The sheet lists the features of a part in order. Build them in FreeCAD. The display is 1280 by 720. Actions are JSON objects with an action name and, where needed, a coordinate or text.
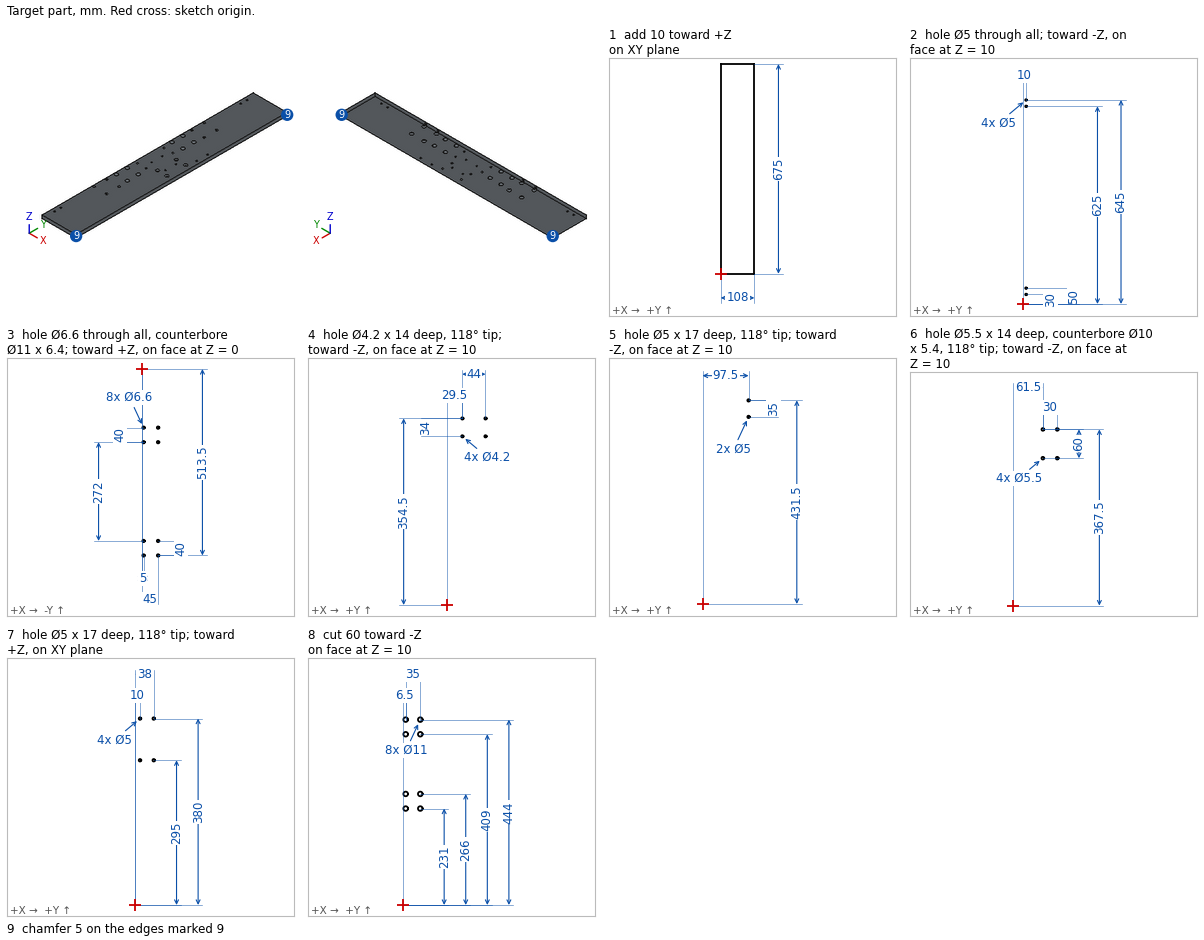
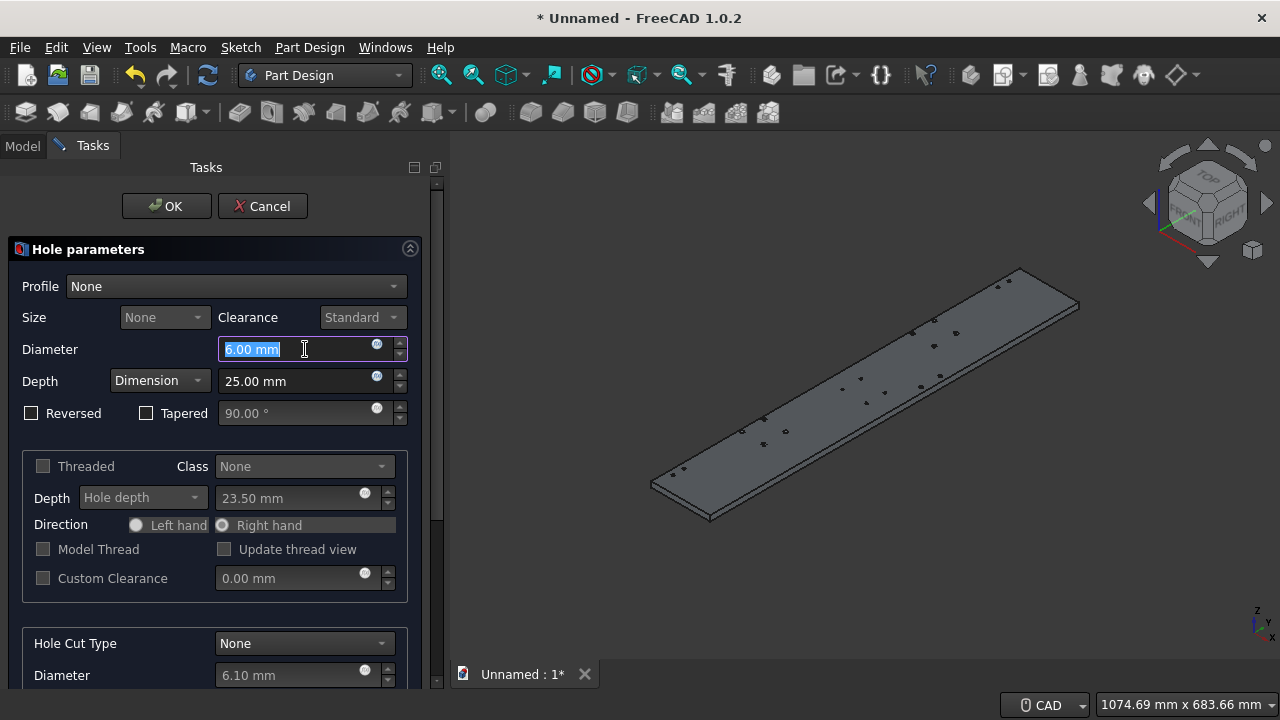
{"action": "type", "text": "5"}
{"action": "key", "text": "Tab"}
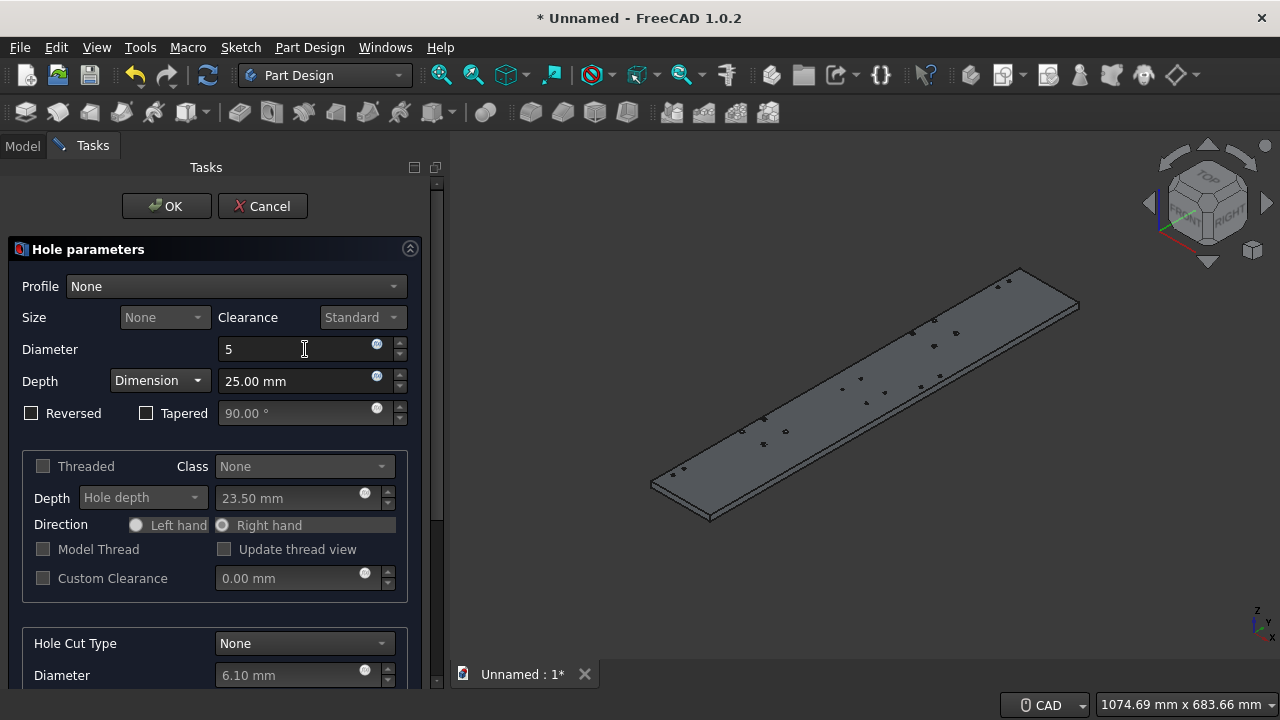
{"action": "triple_click", "coordinate": [305, 381]}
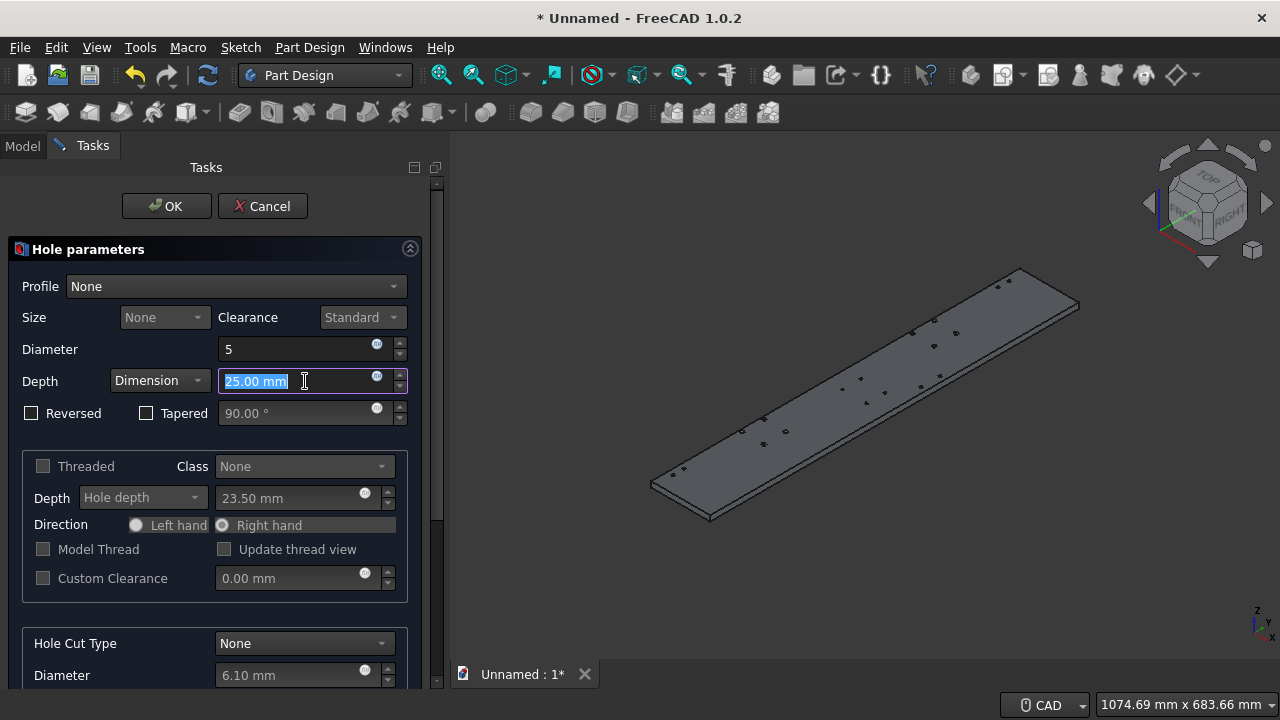
{"action": "type", "text": "17"}
{"action": "key", "text": "Tab"}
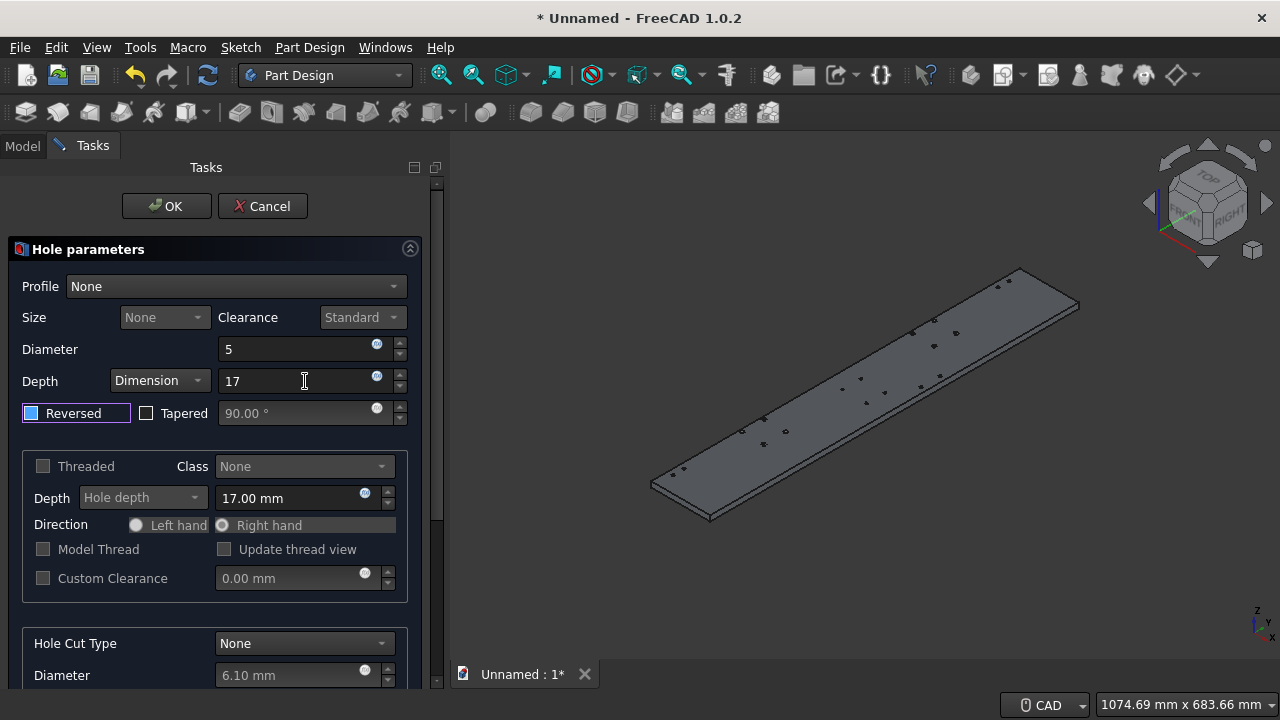
{"action": "left_click", "coordinate": [167, 206]}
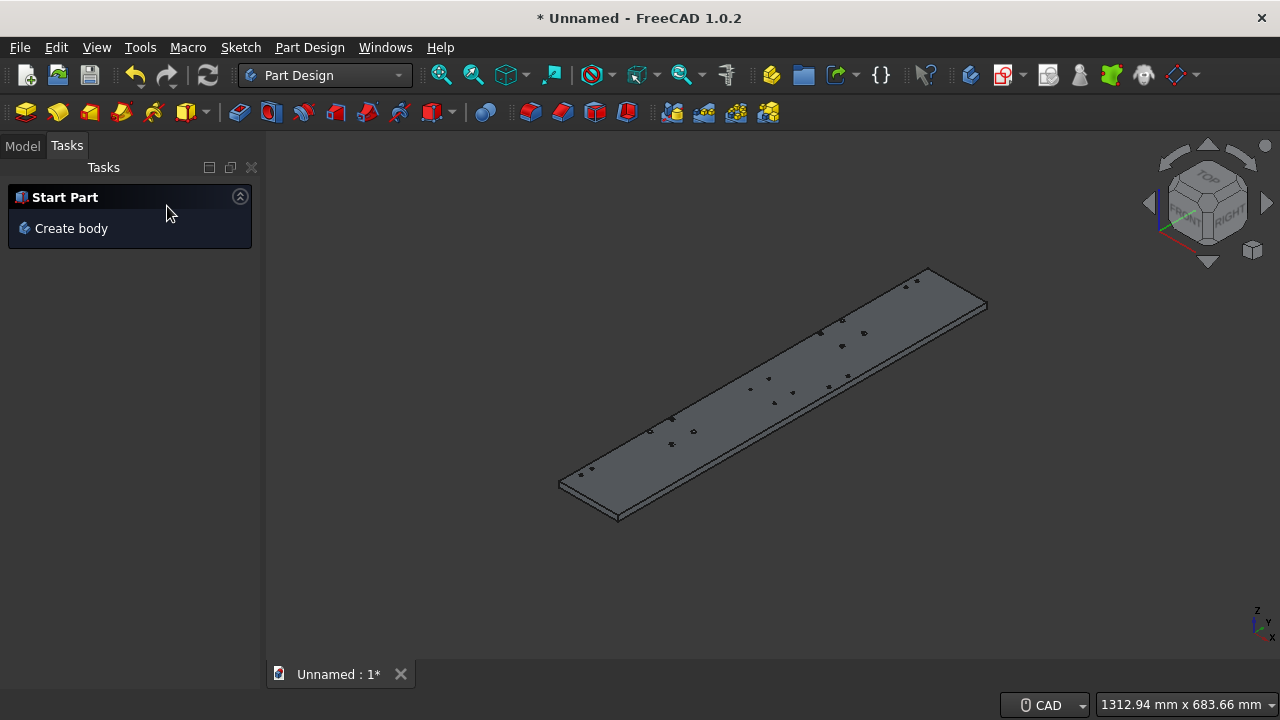
{"action": "left_click", "coordinate": [931, 300]}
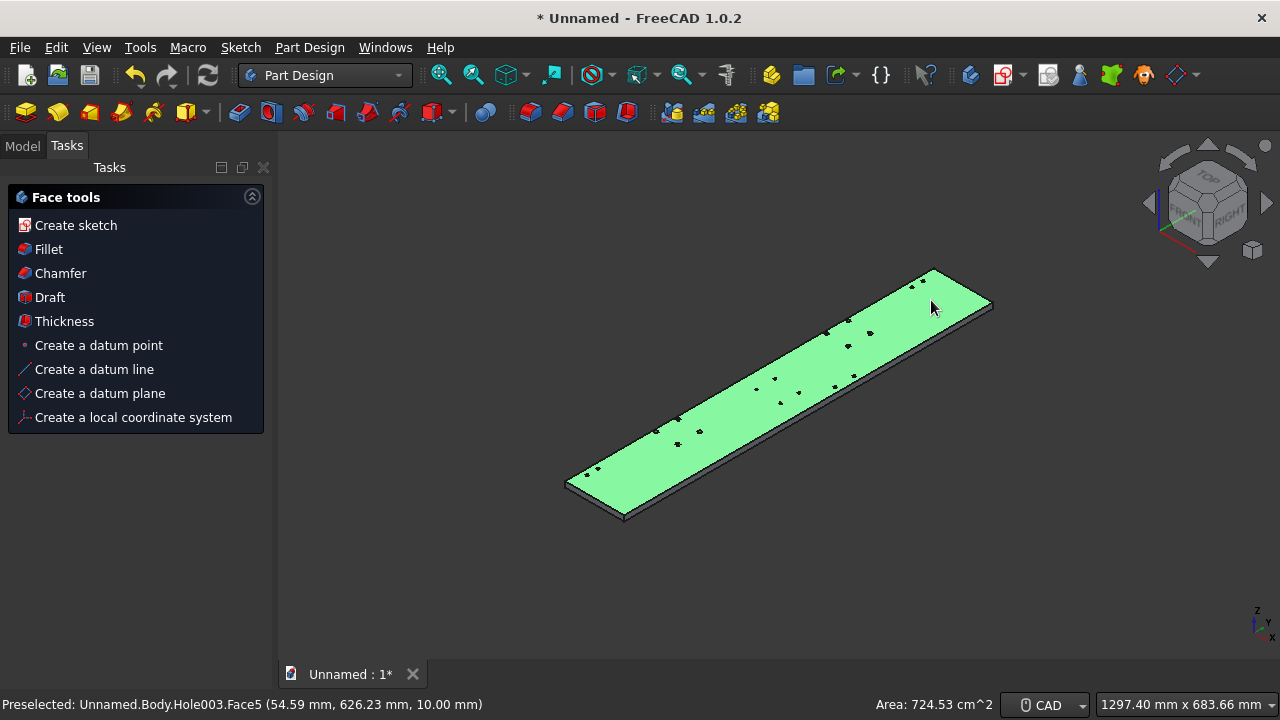
{"action": "left_click", "coordinate": [1004, 76]}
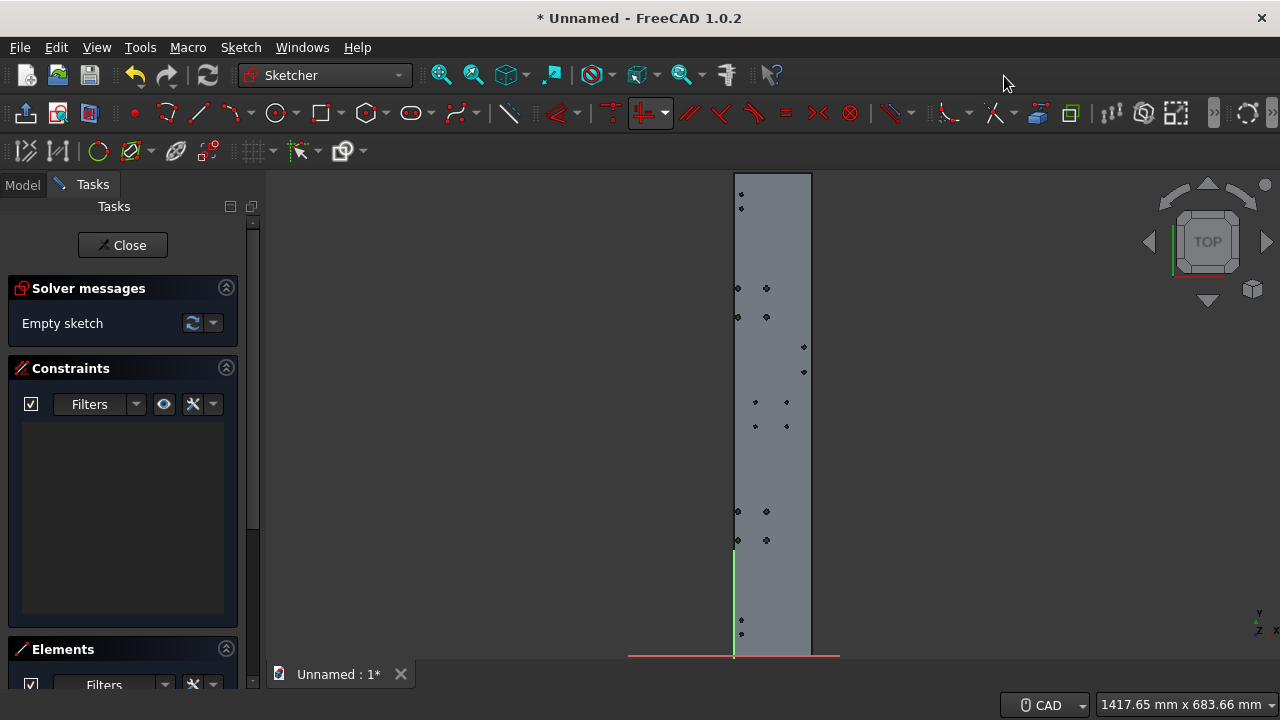
{"action": "scroll", "coordinate": [806, 414], "scroll_direction": "up", "scroll_amount": 9}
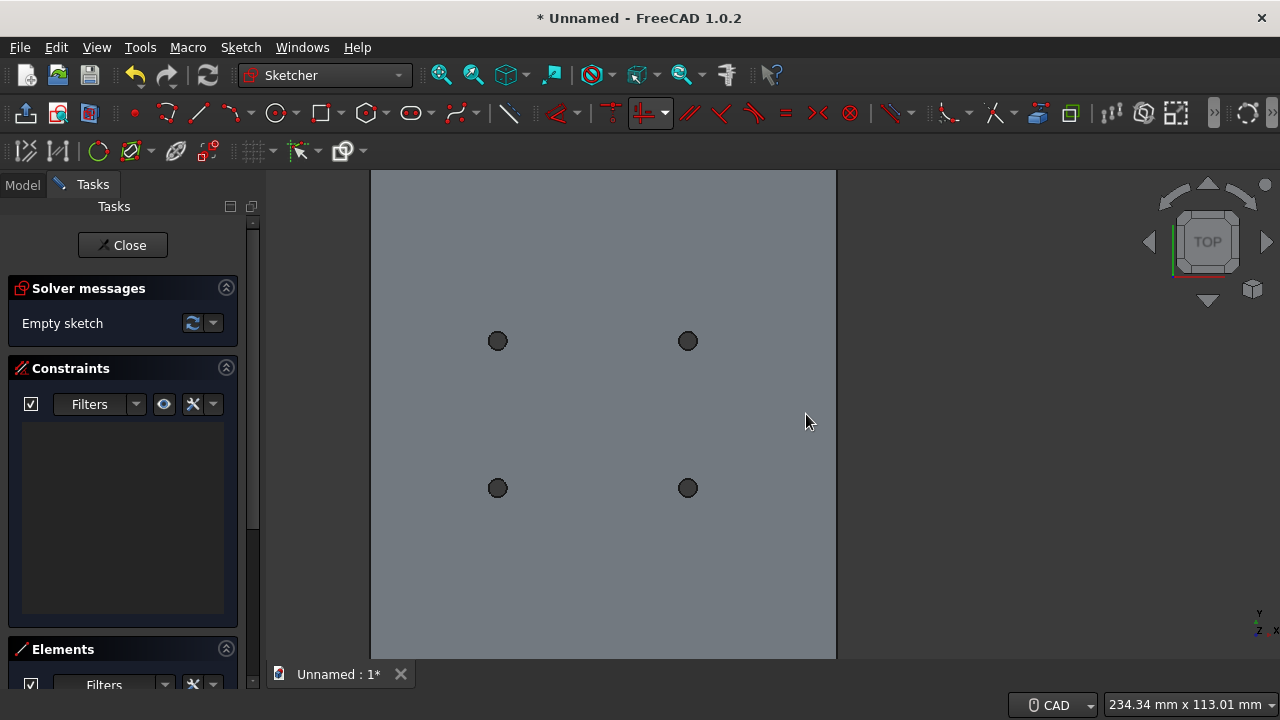
{"action": "left_click", "coordinate": [276, 114]}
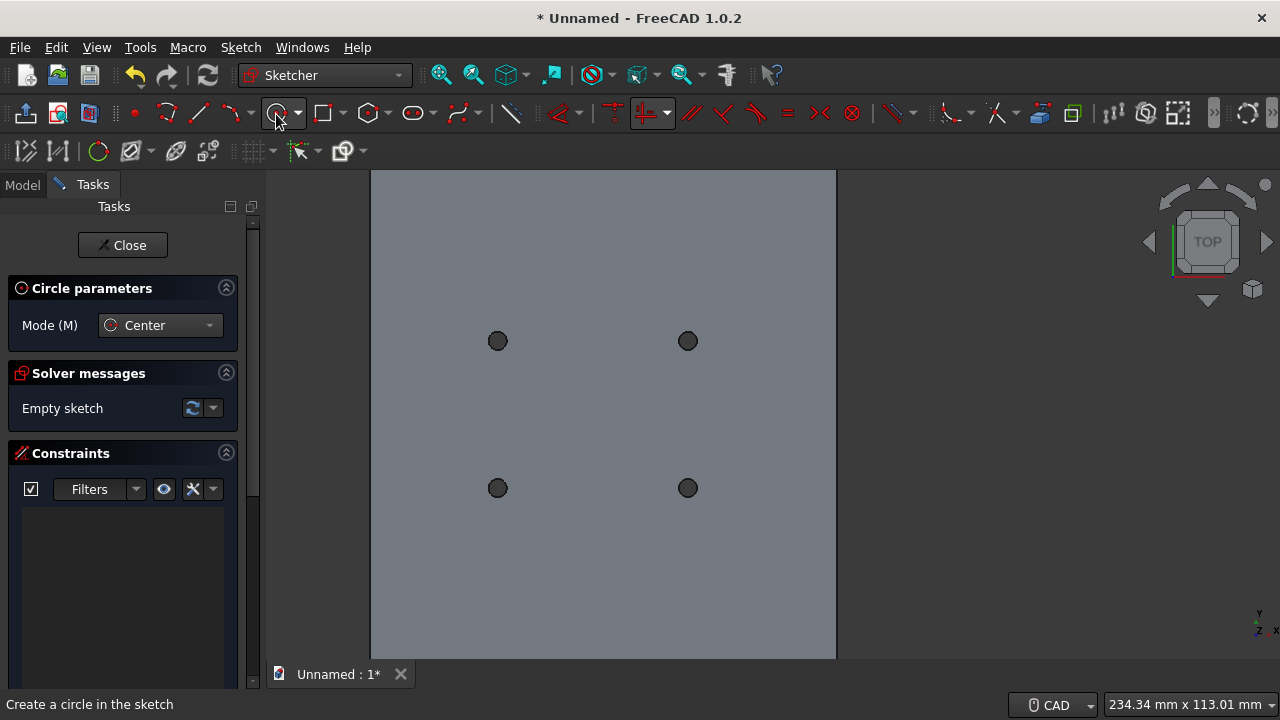
{"action": "scroll", "coordinate": [636, 285], "scroll_direction": "up", "scroll_amount": 4}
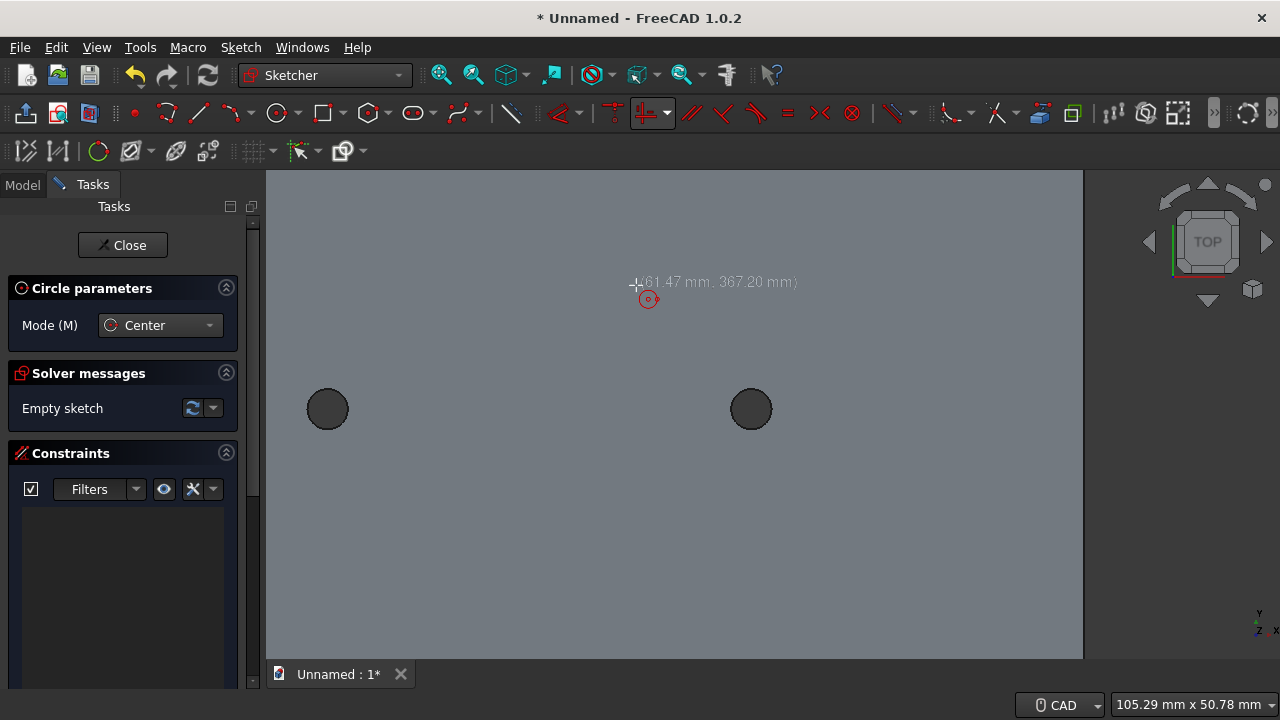
{"action": "left_click", "coordinate": [636, 284]}
{"action": "mouse_move", "coordinate": [655, 265]}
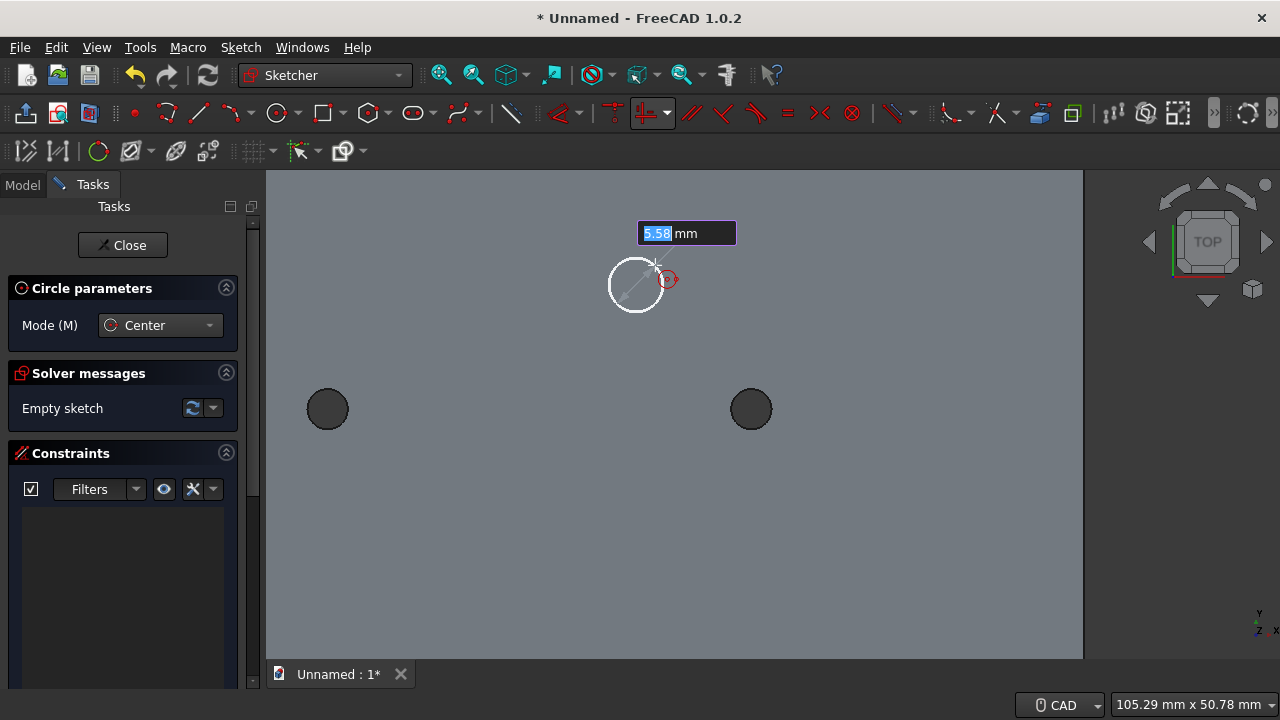
{"action": "type", "text": "5.5"}
{"action": "key", "text": "Return"}